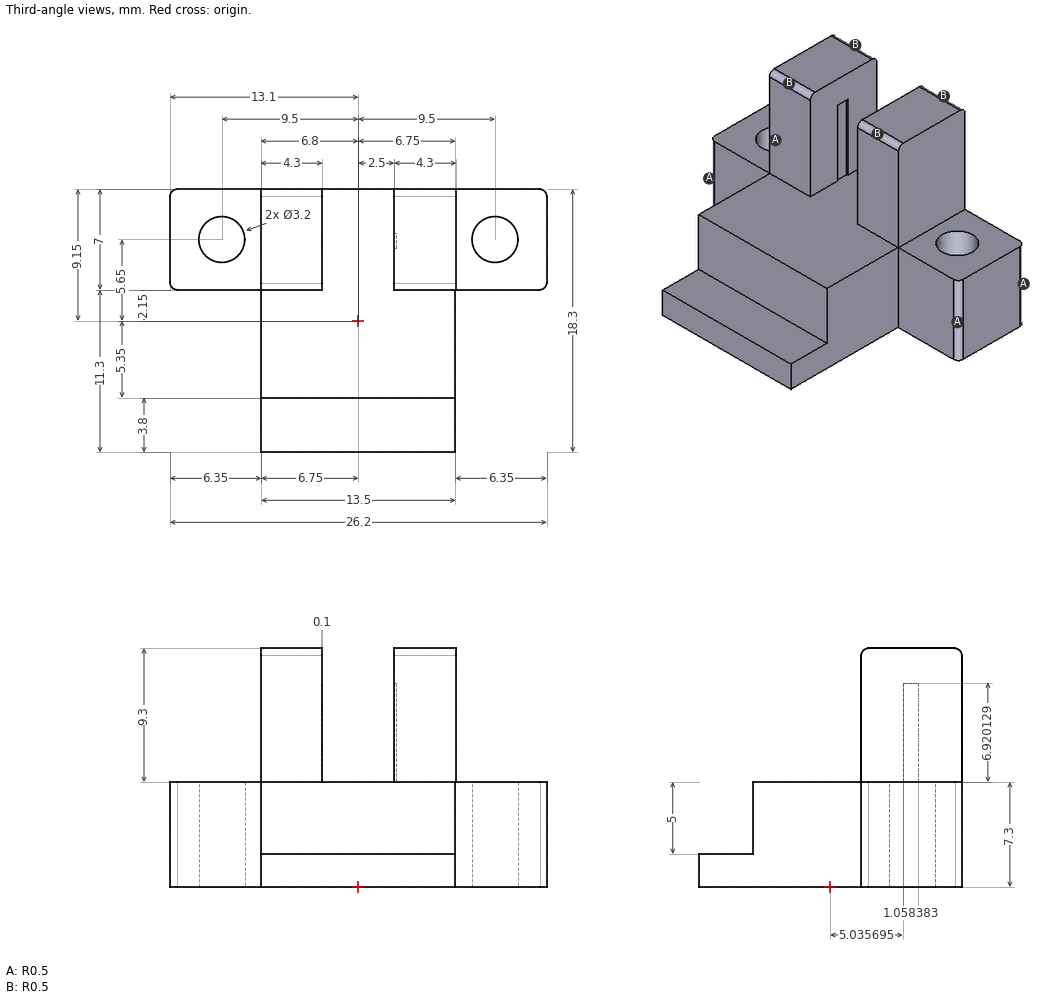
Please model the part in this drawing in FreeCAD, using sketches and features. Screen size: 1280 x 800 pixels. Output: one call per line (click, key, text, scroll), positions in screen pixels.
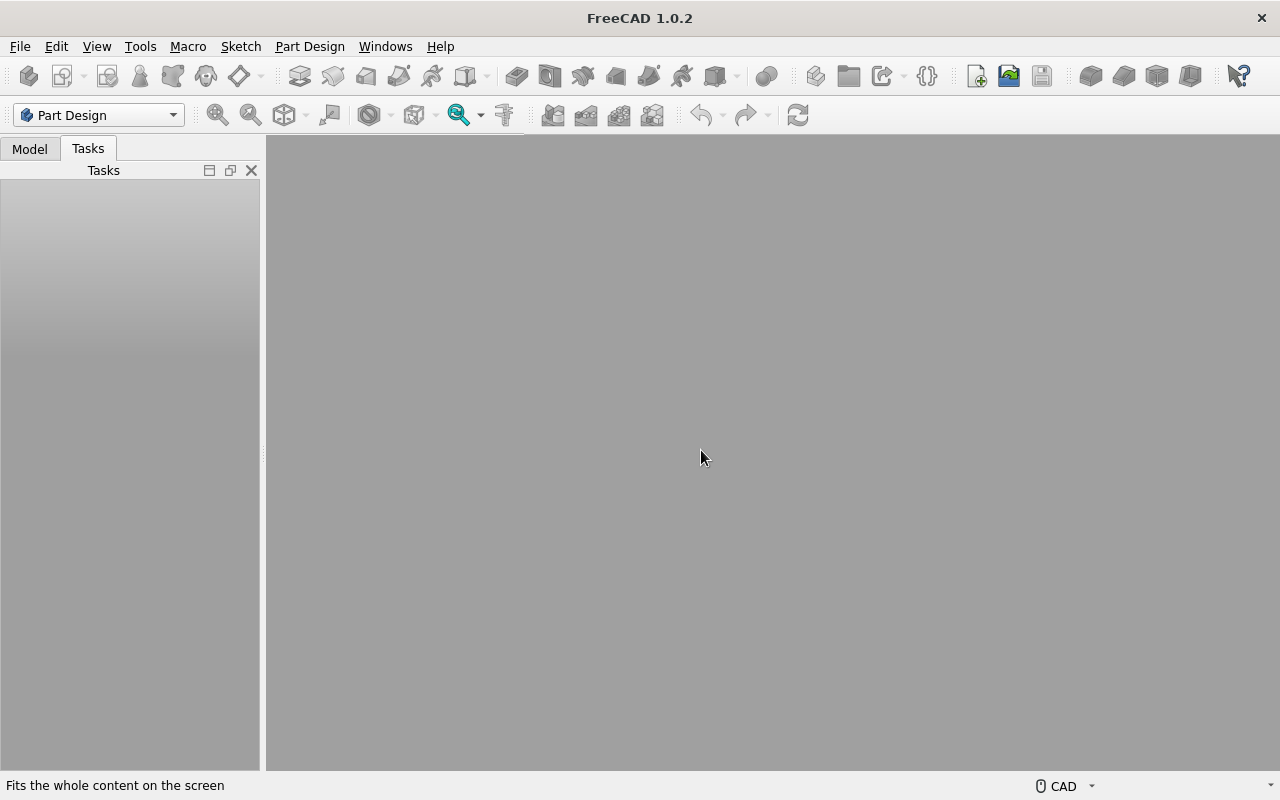
key(ctrl+n)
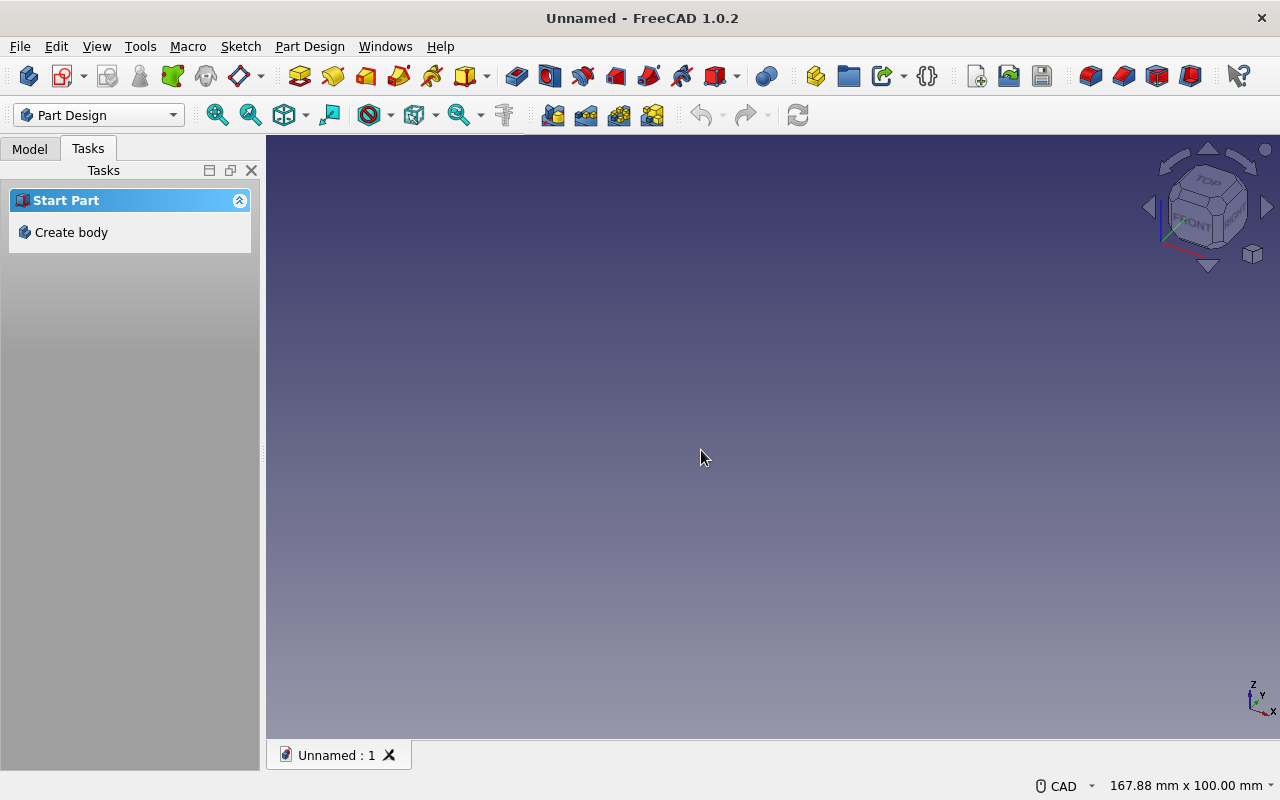
click(62, 76)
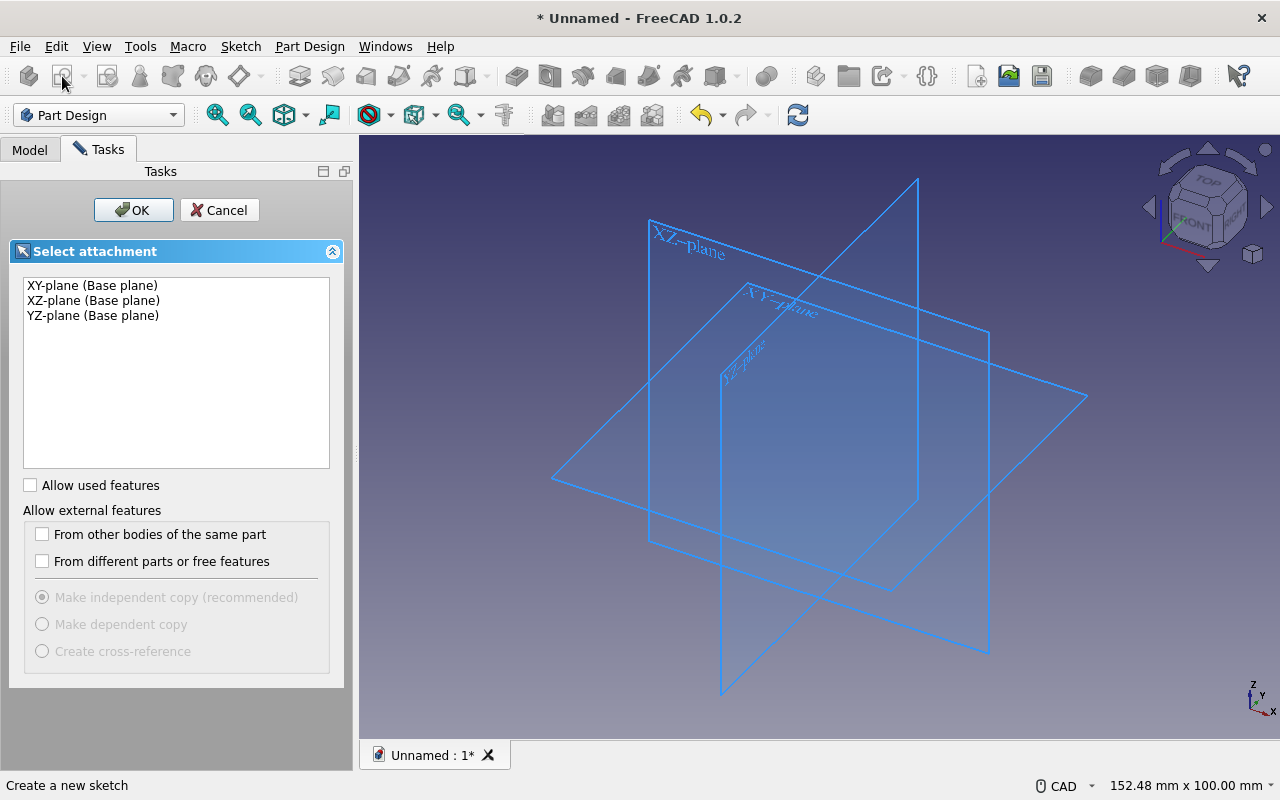
click(84, 286)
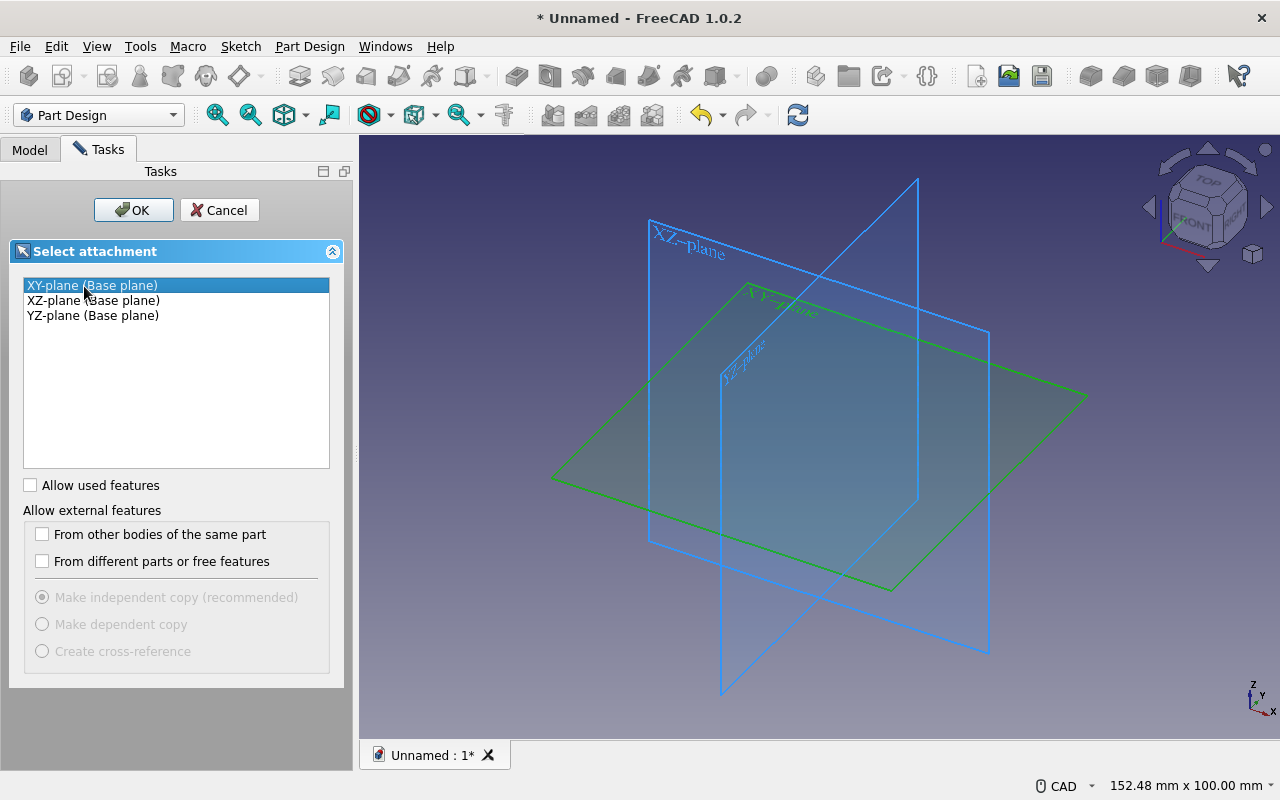
click(134, 210)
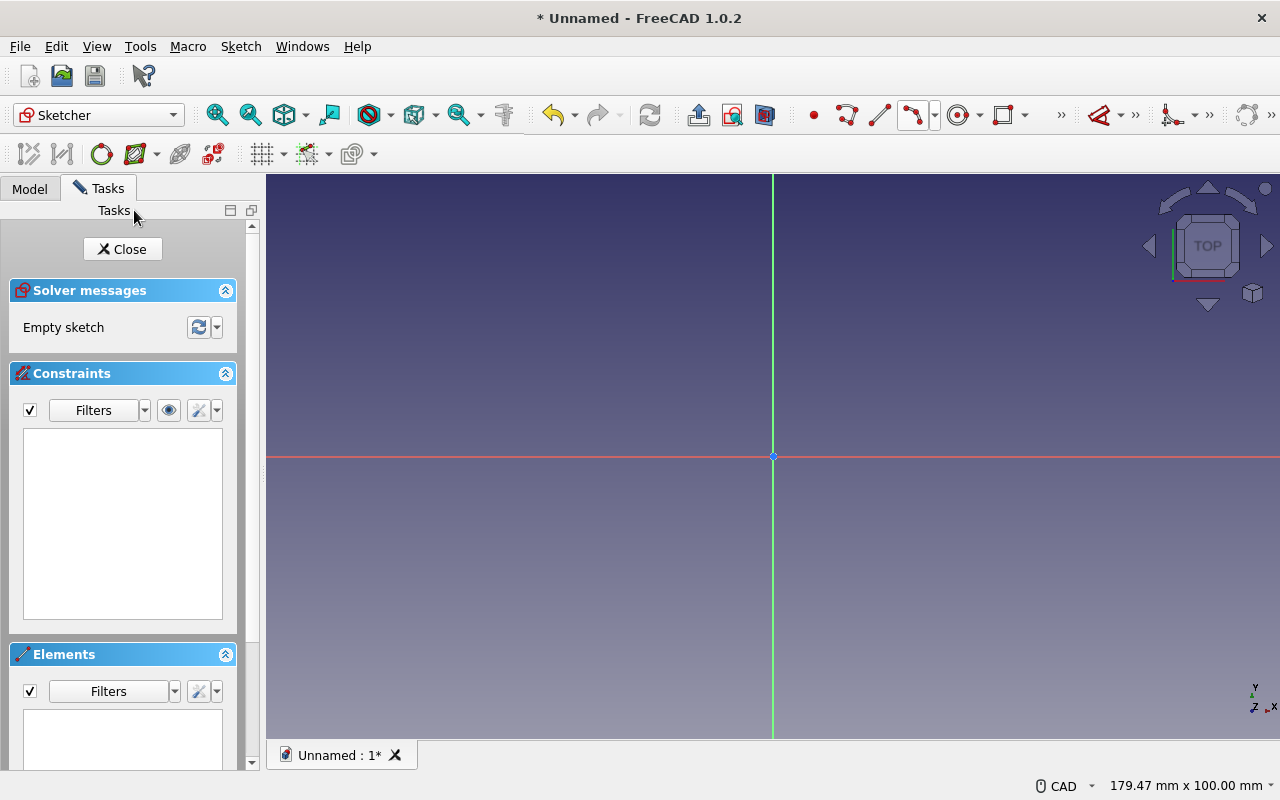
scroll(803, 456, up, 6)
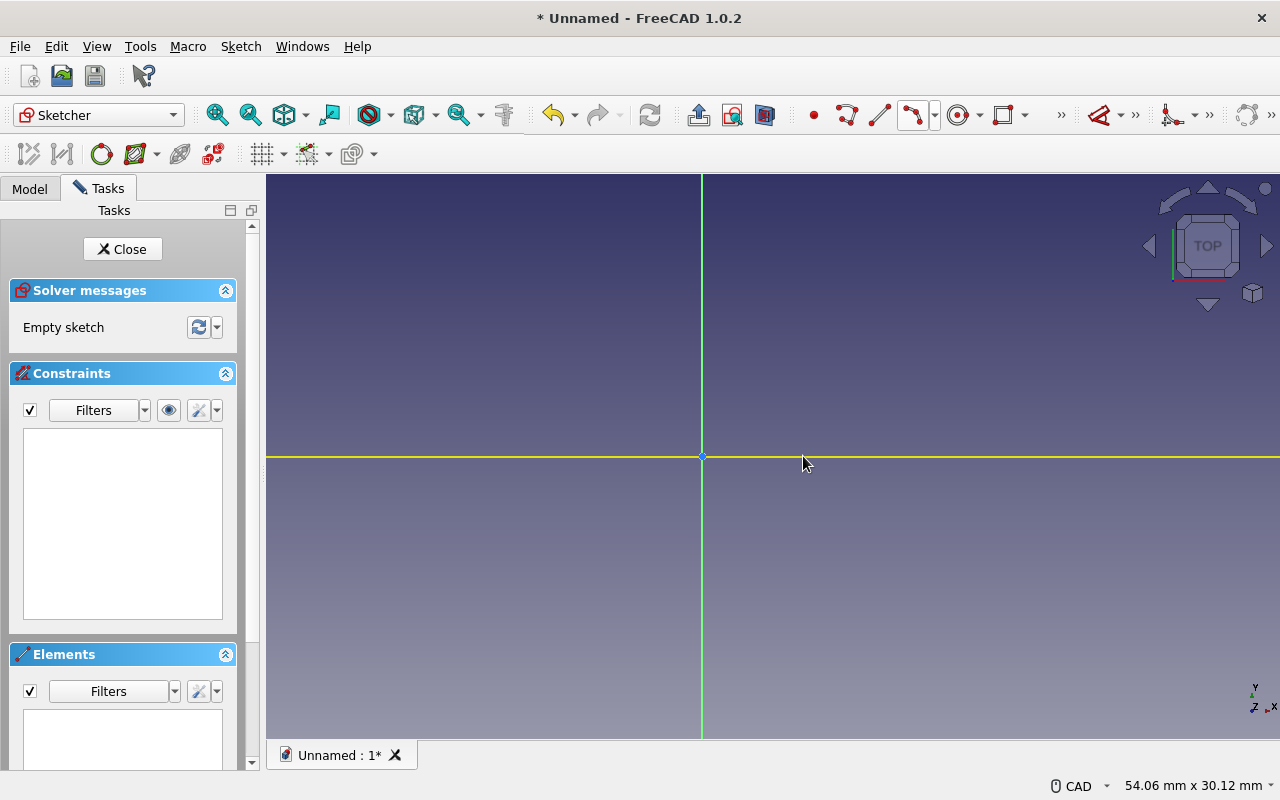
key(g)
key(v)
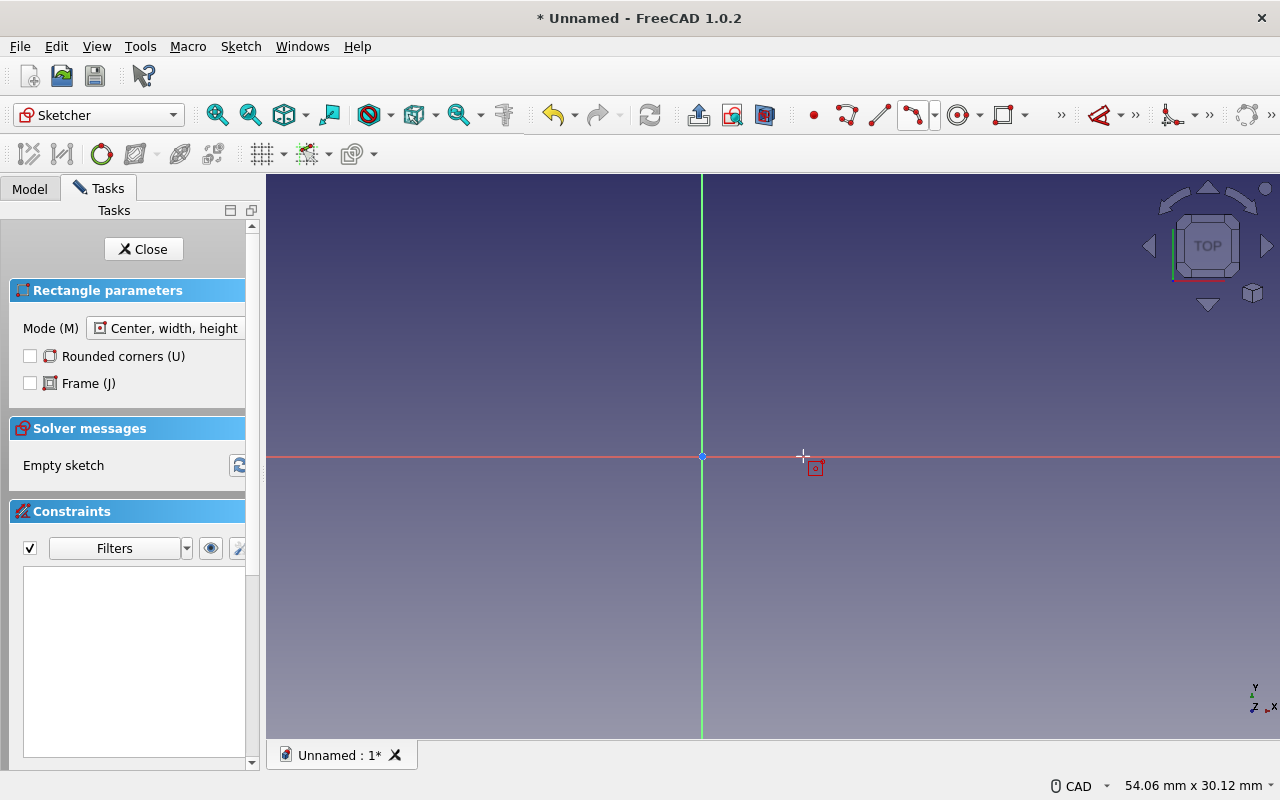
click(702, 456)
click(948, 285)
key(Escape)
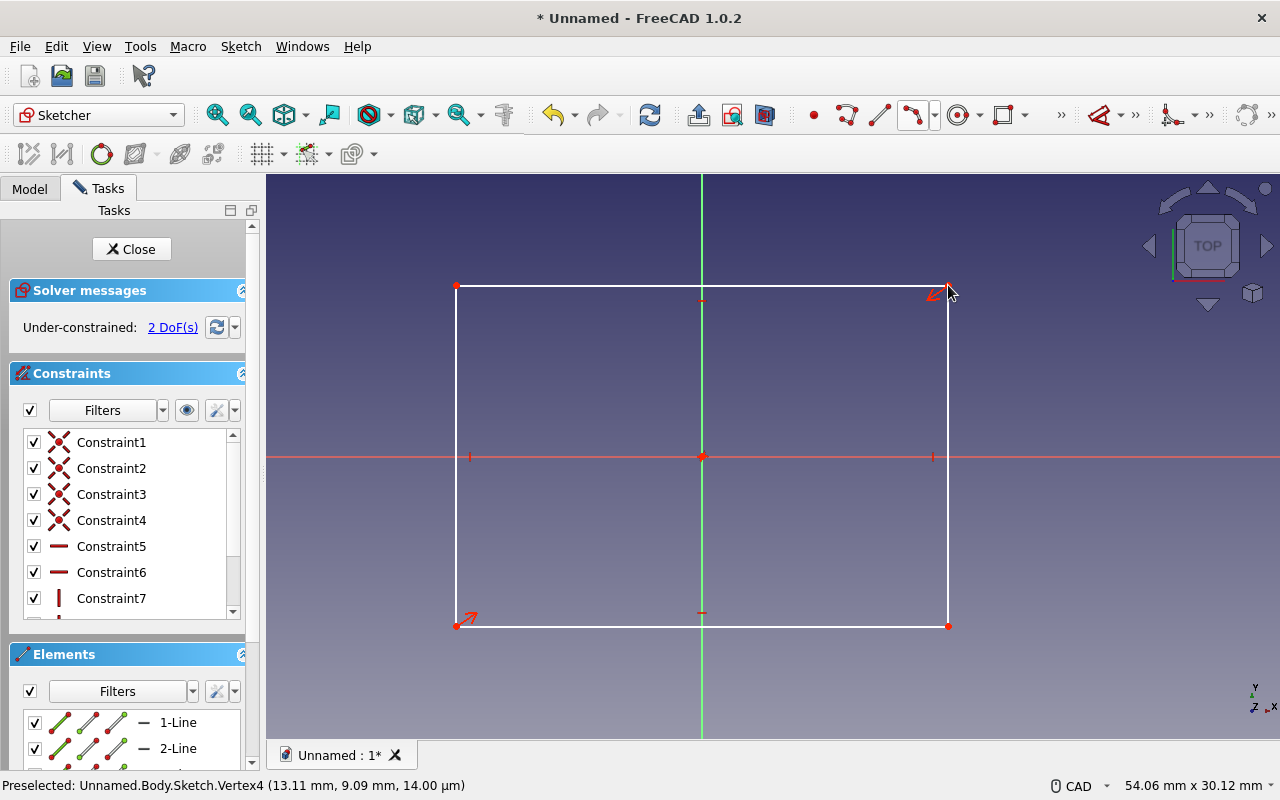
click(604, 627)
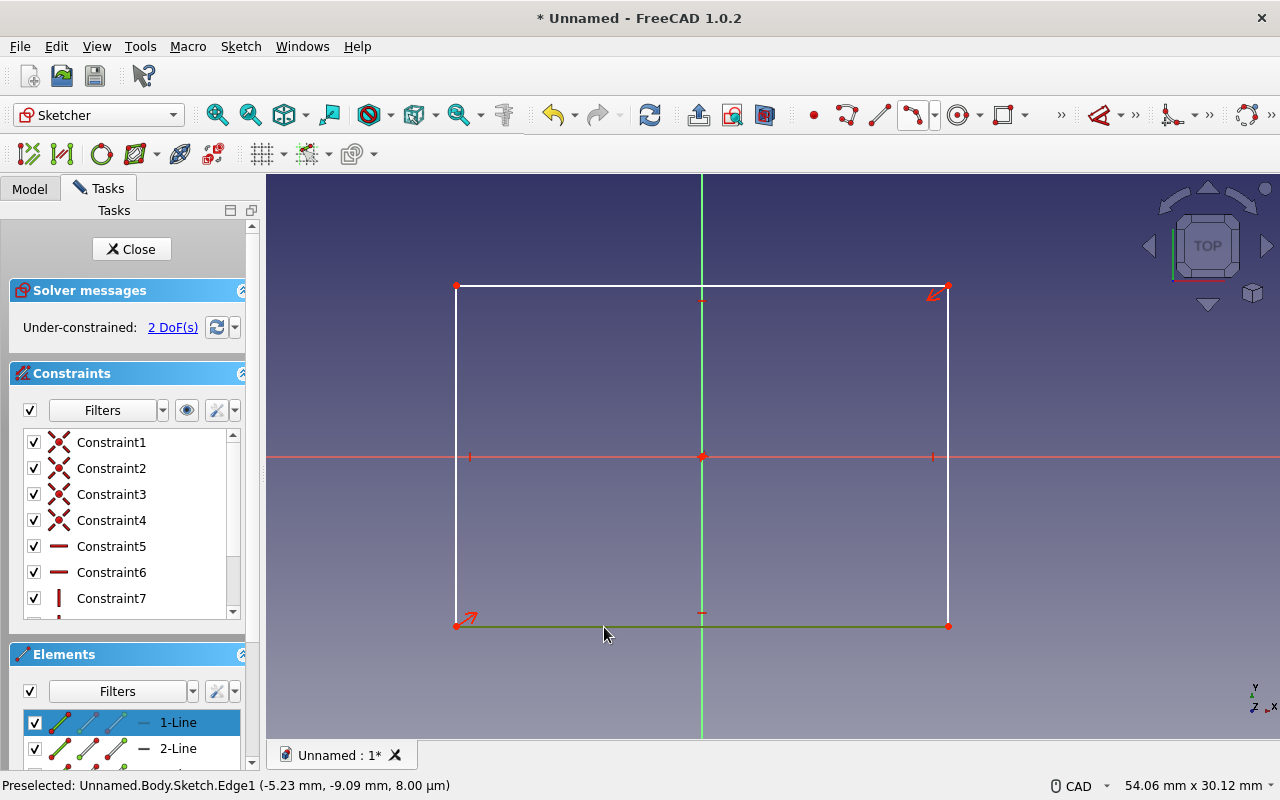
key(l)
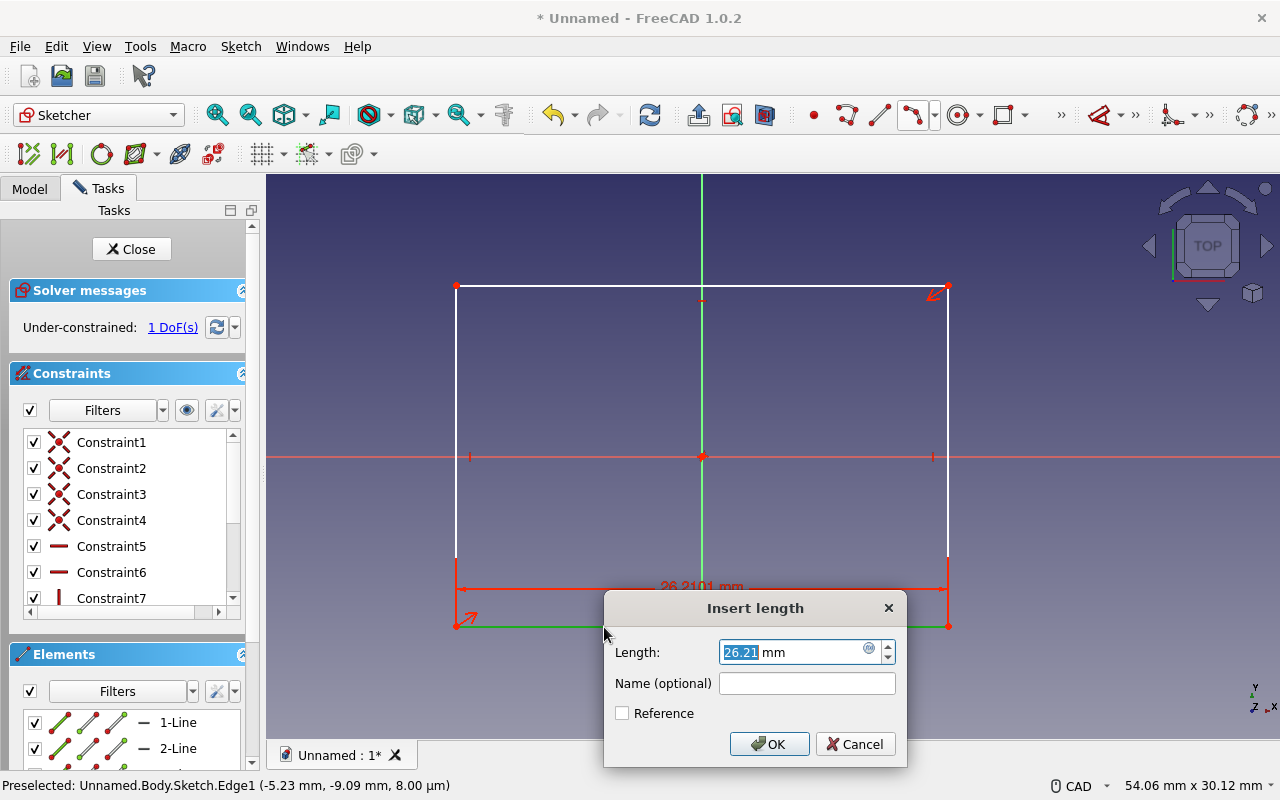
text(26.2)
key(Return)